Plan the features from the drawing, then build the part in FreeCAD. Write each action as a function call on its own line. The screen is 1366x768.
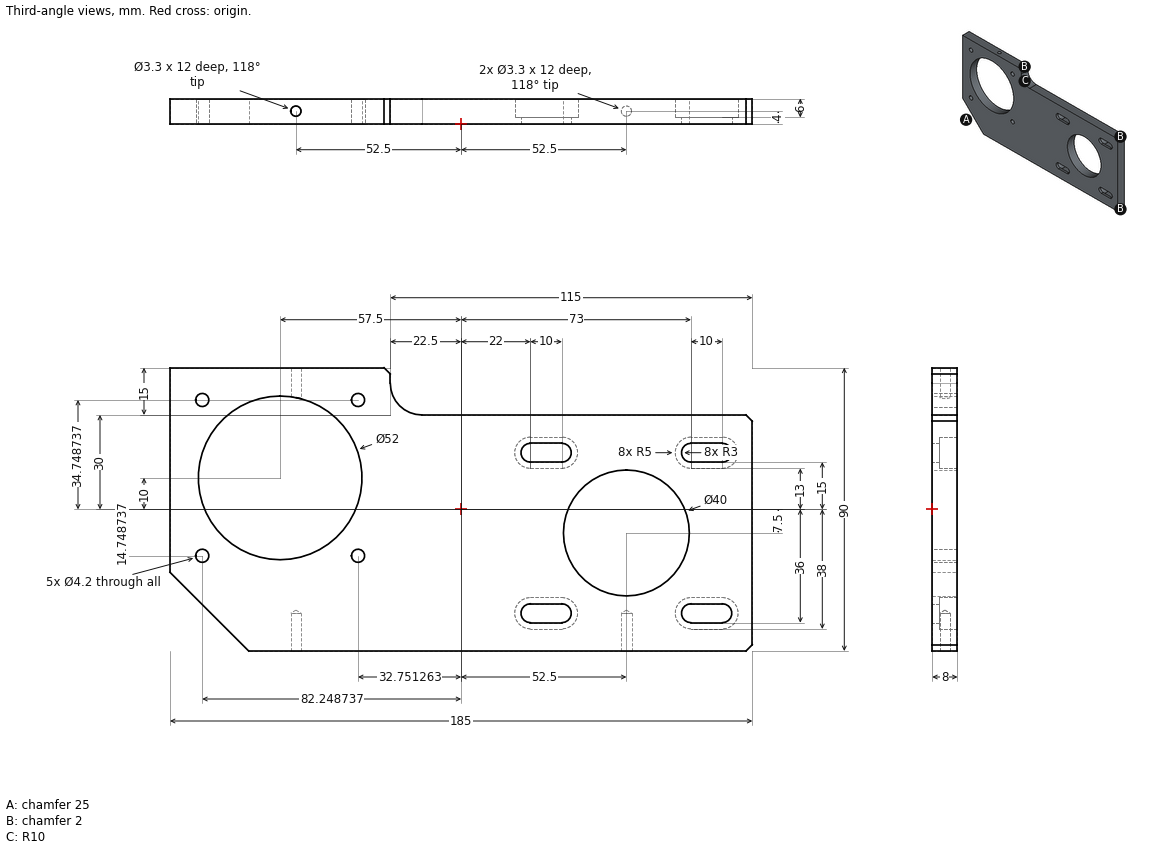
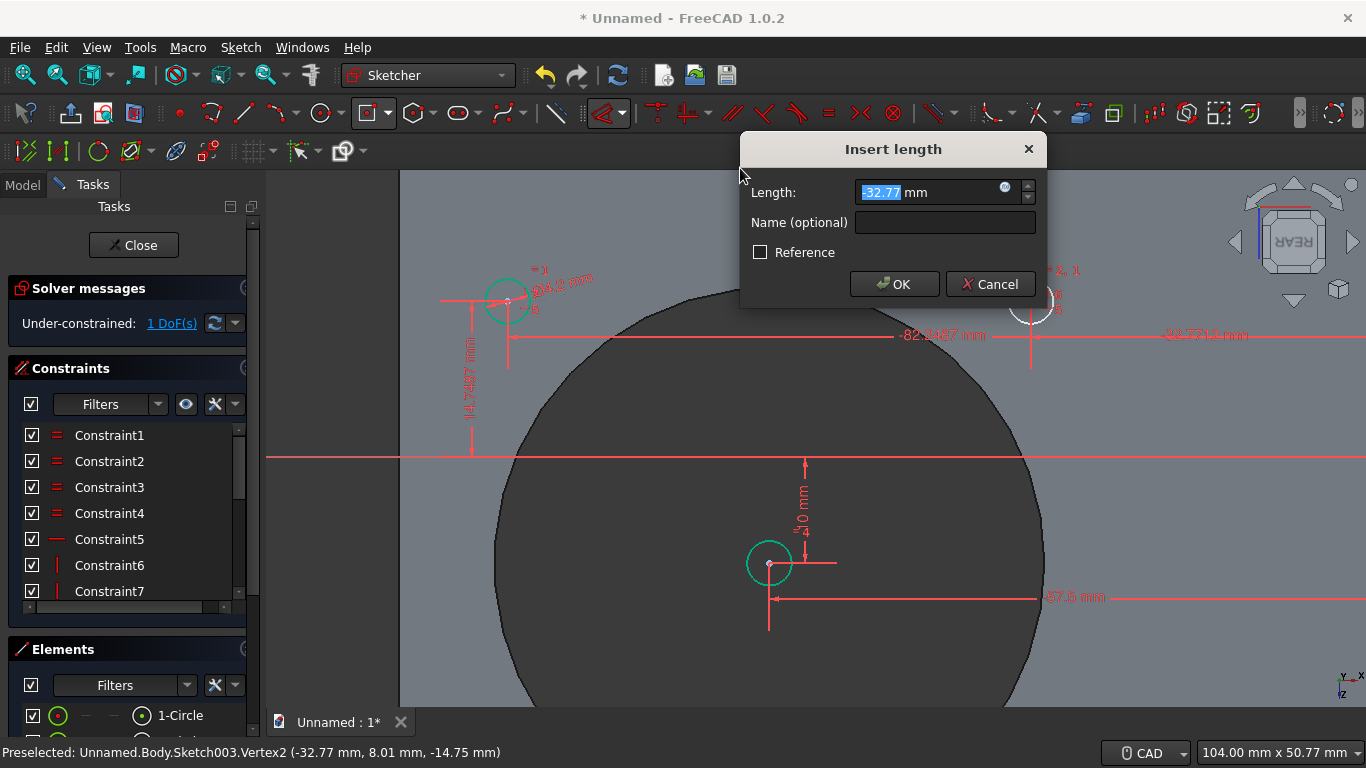
text(-32.751263)
key(Return)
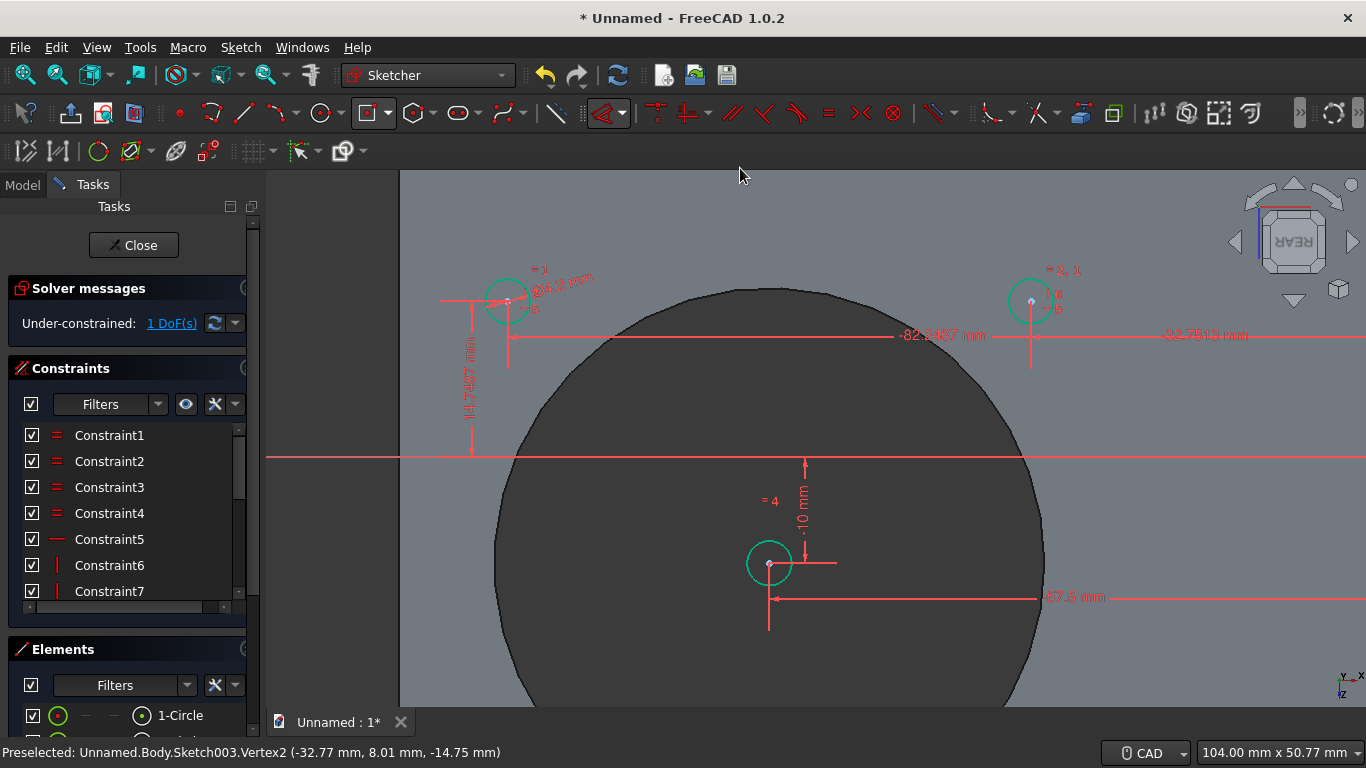
scroll(524, 287, down, 3)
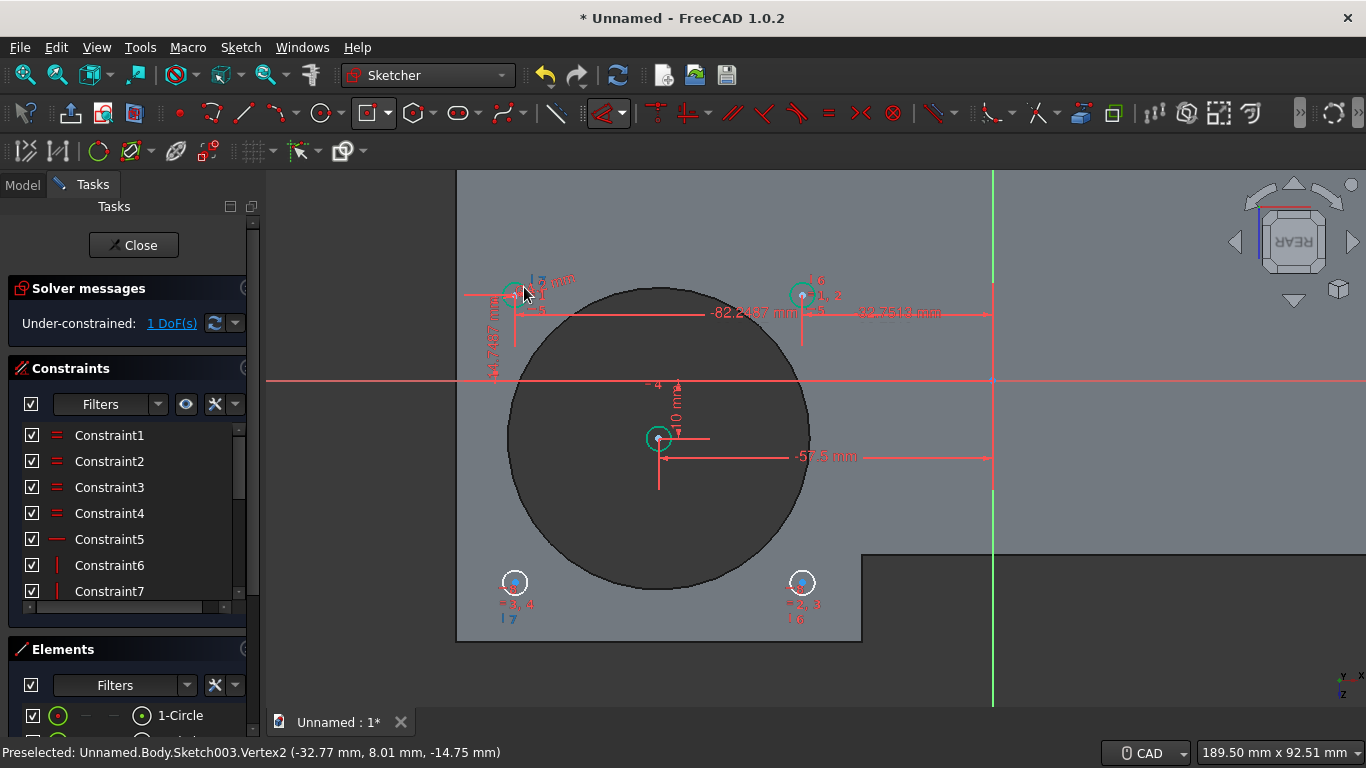
click(802, 583)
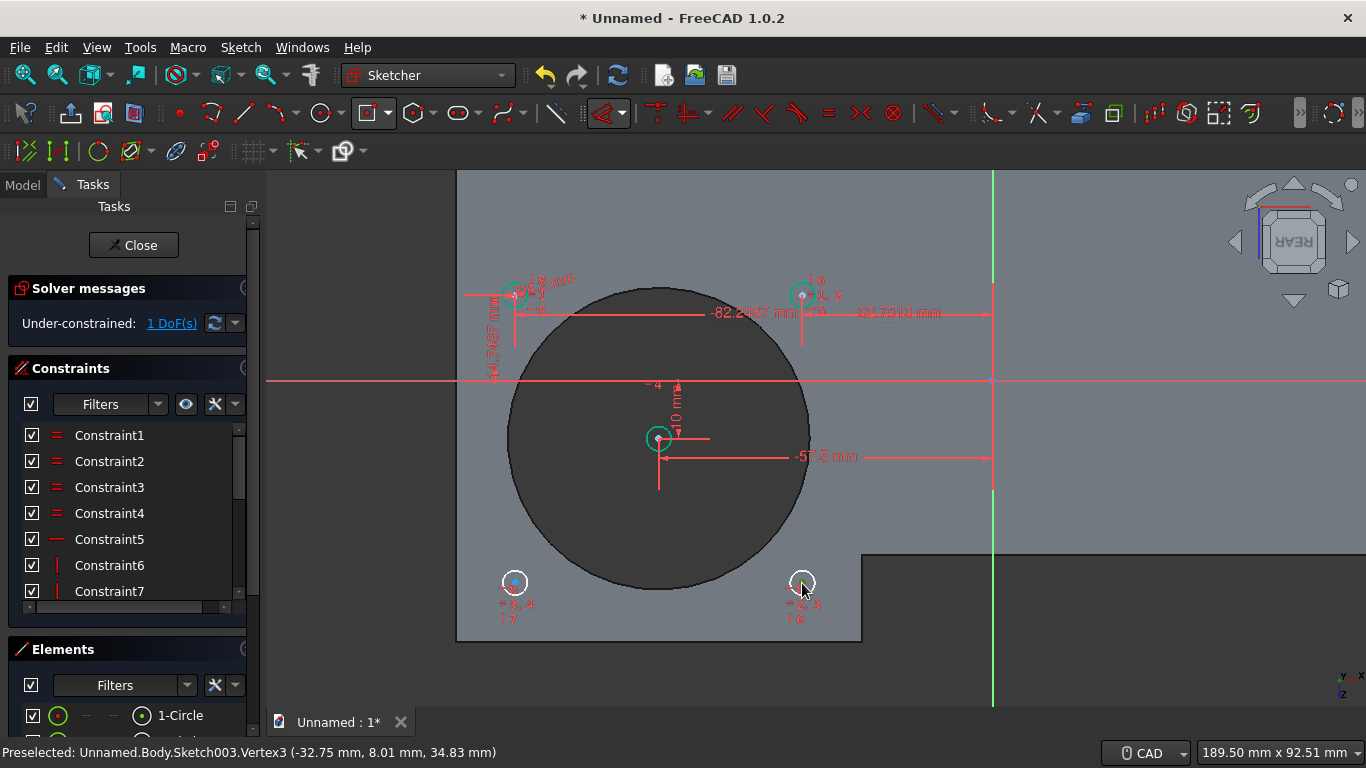
click(624, 114)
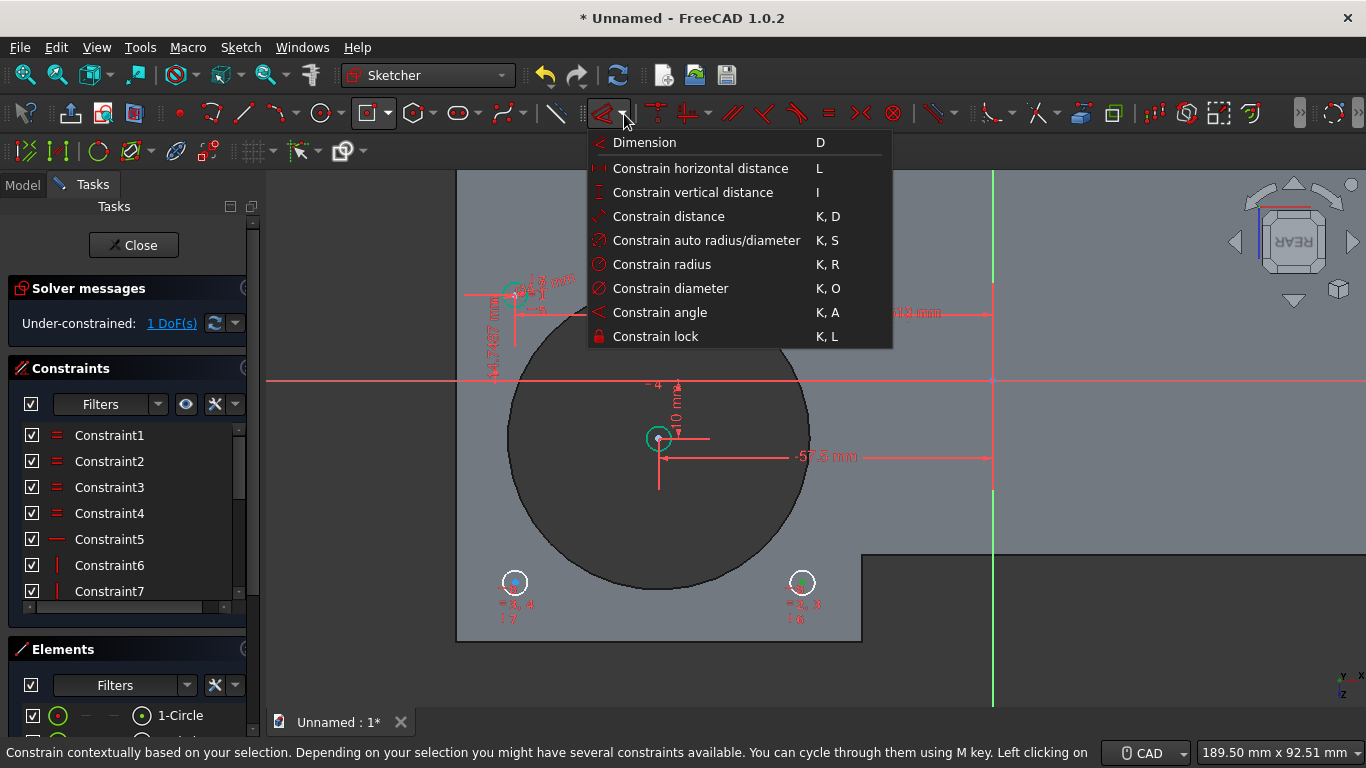
click(740, 192)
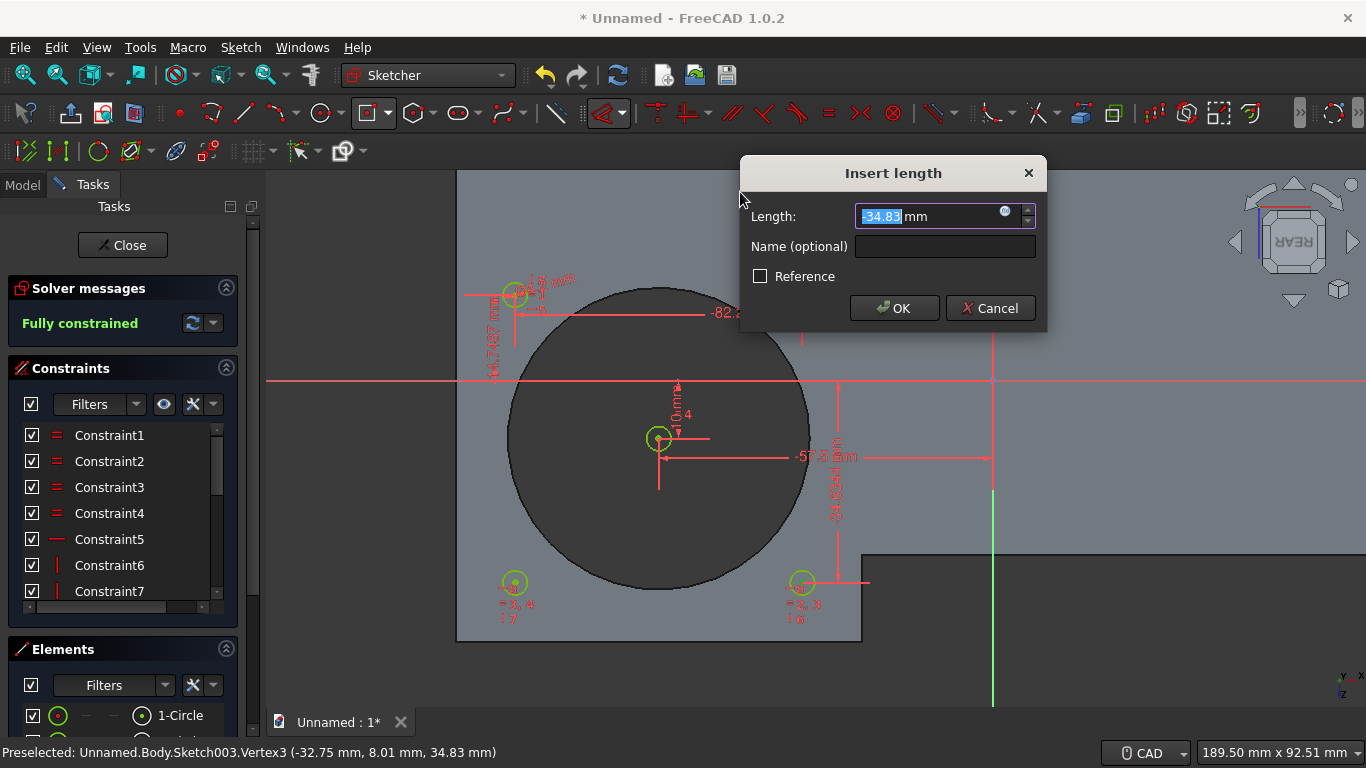
text(-34.748737)
key(Return)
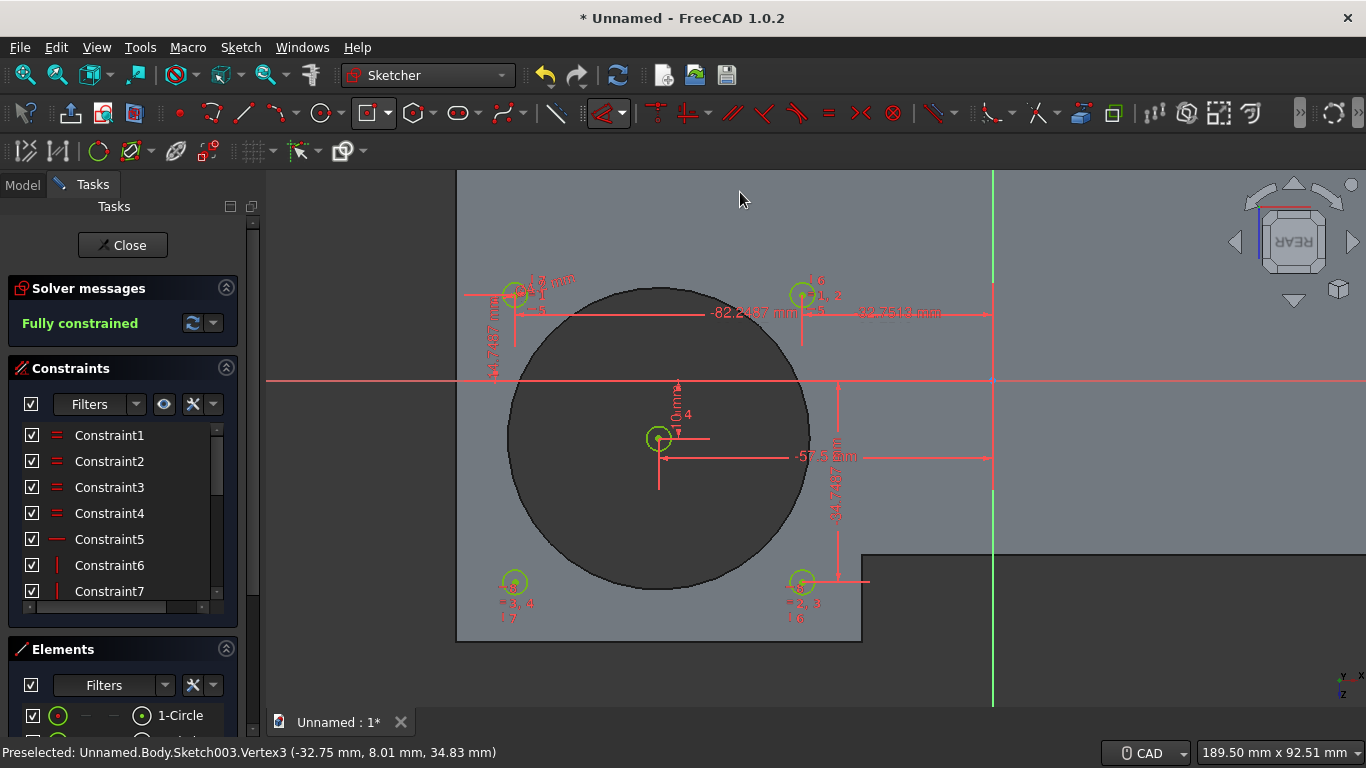
click(123, 245)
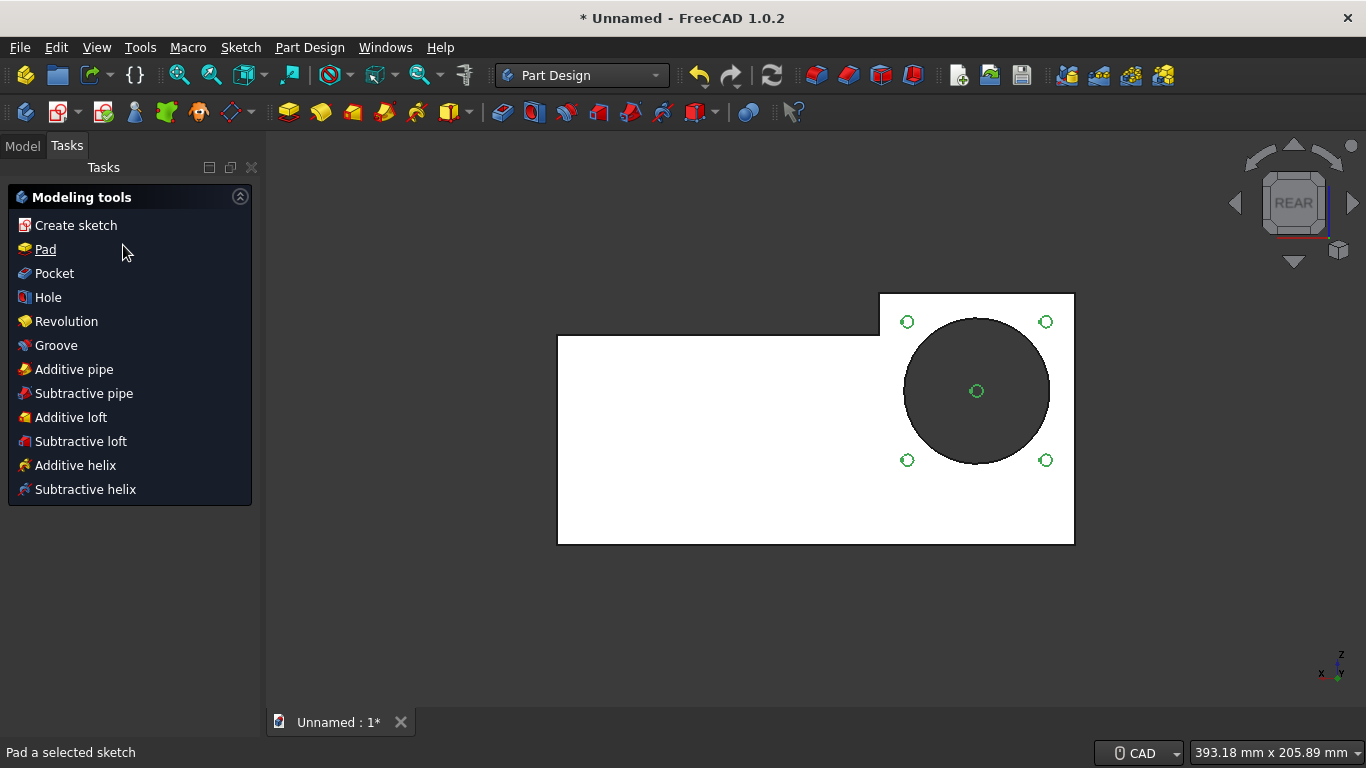
click(536, 112)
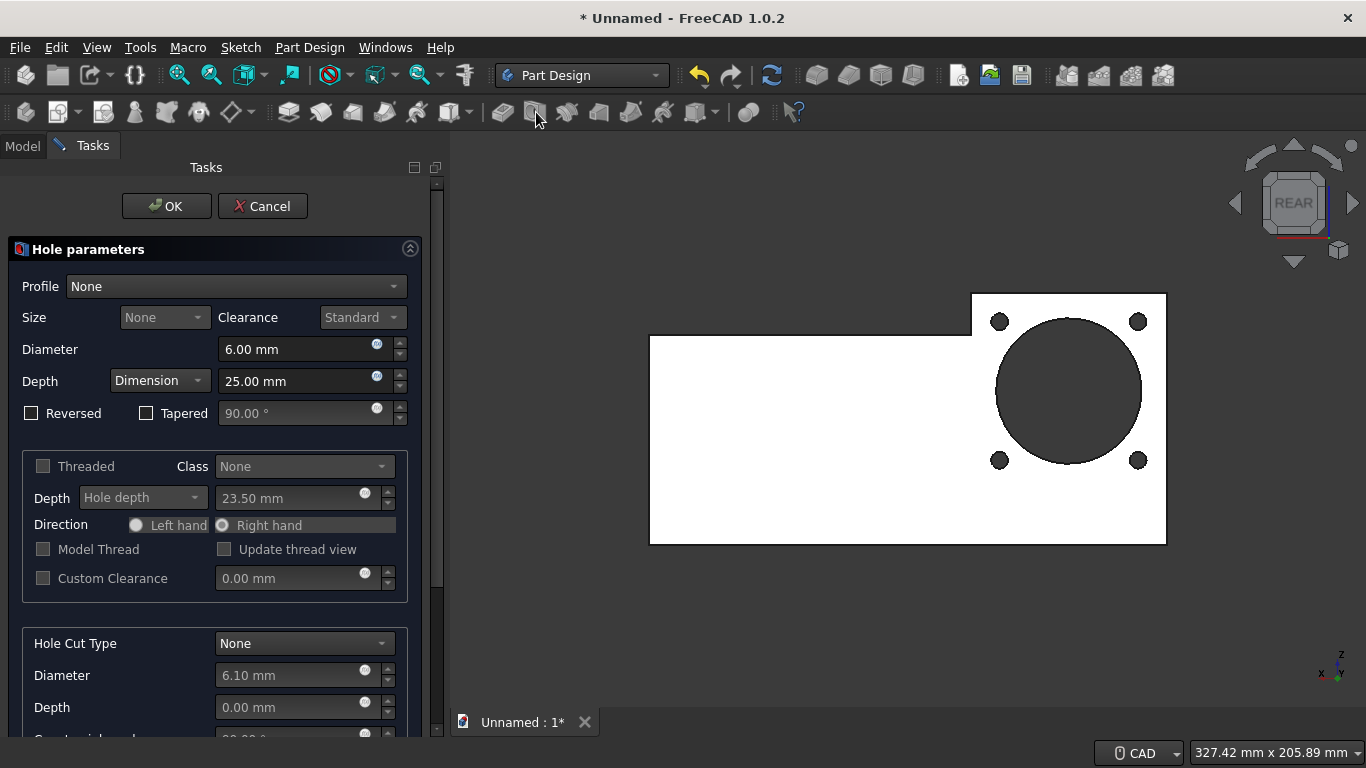
triple_click(305, 349)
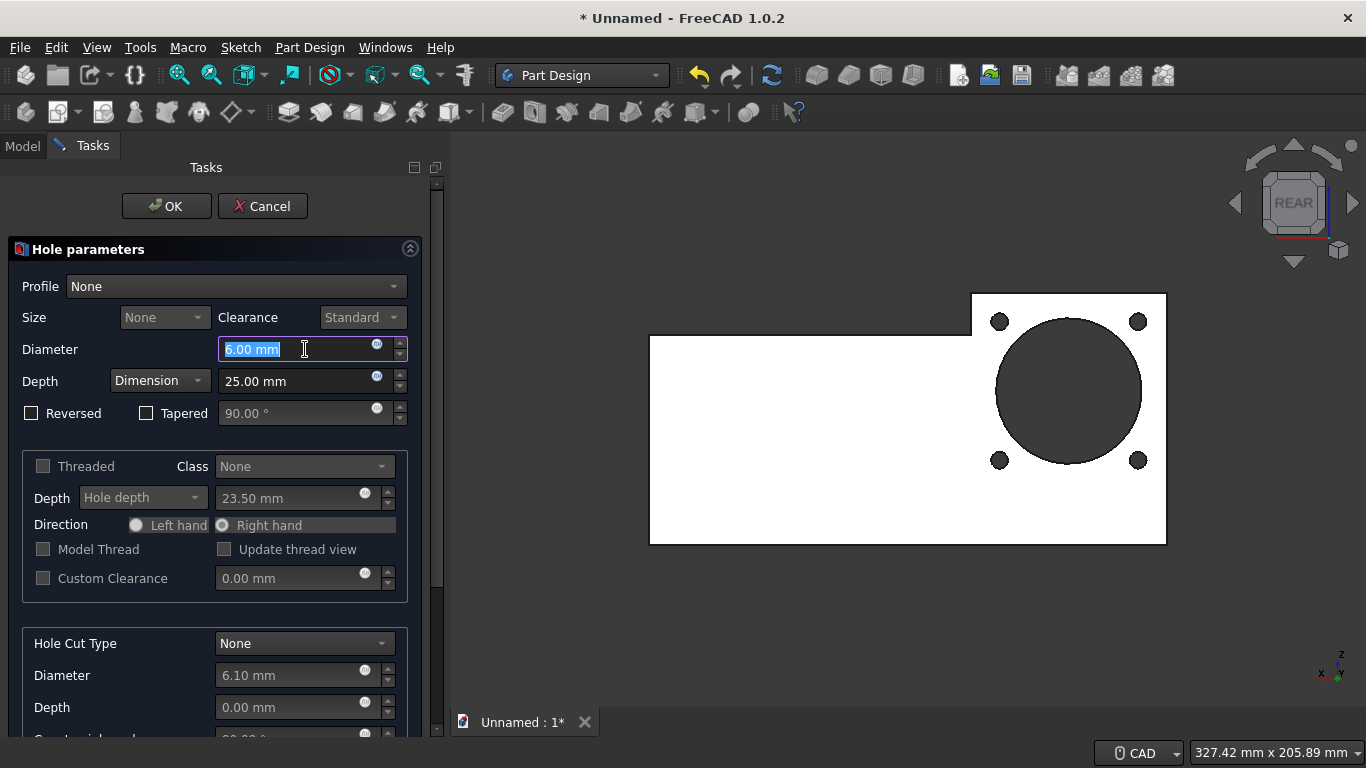
text(4.2)
key(Tab)